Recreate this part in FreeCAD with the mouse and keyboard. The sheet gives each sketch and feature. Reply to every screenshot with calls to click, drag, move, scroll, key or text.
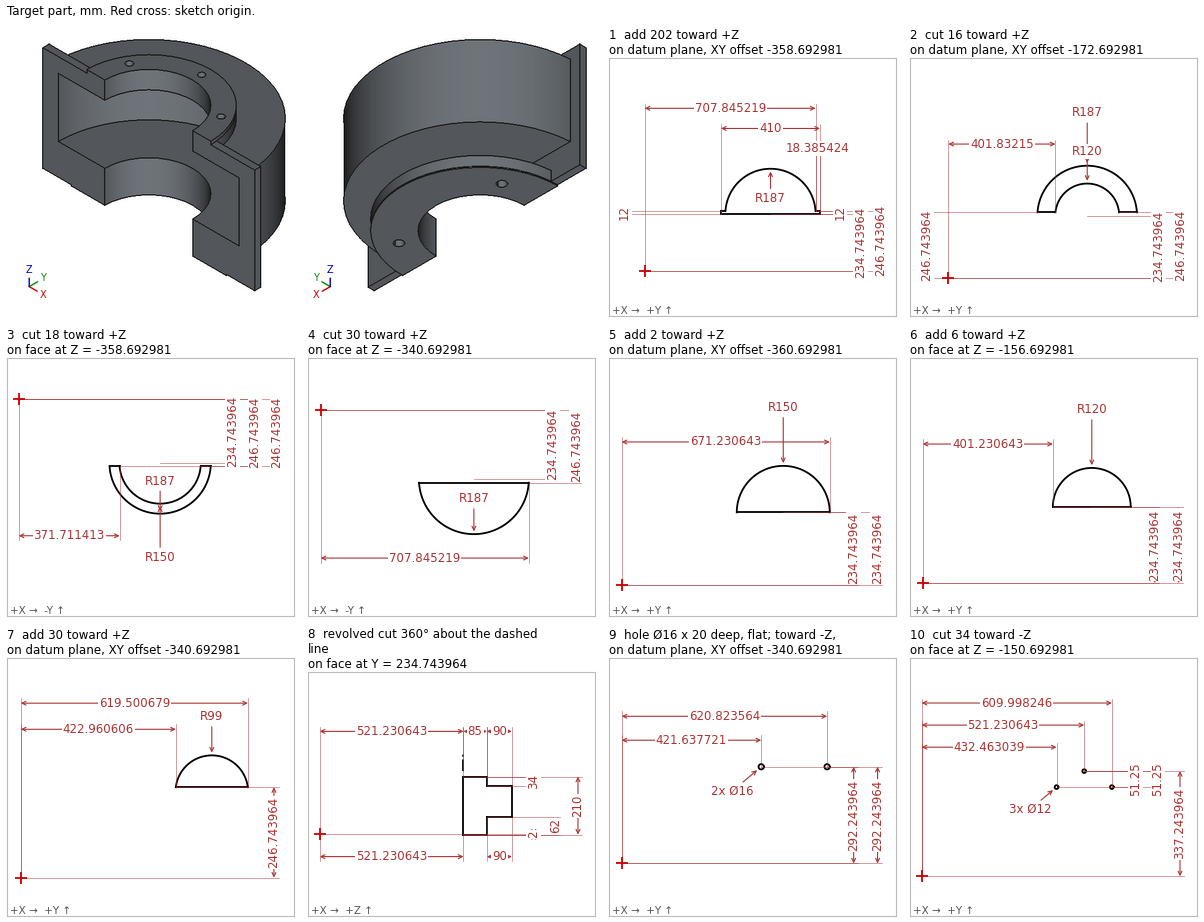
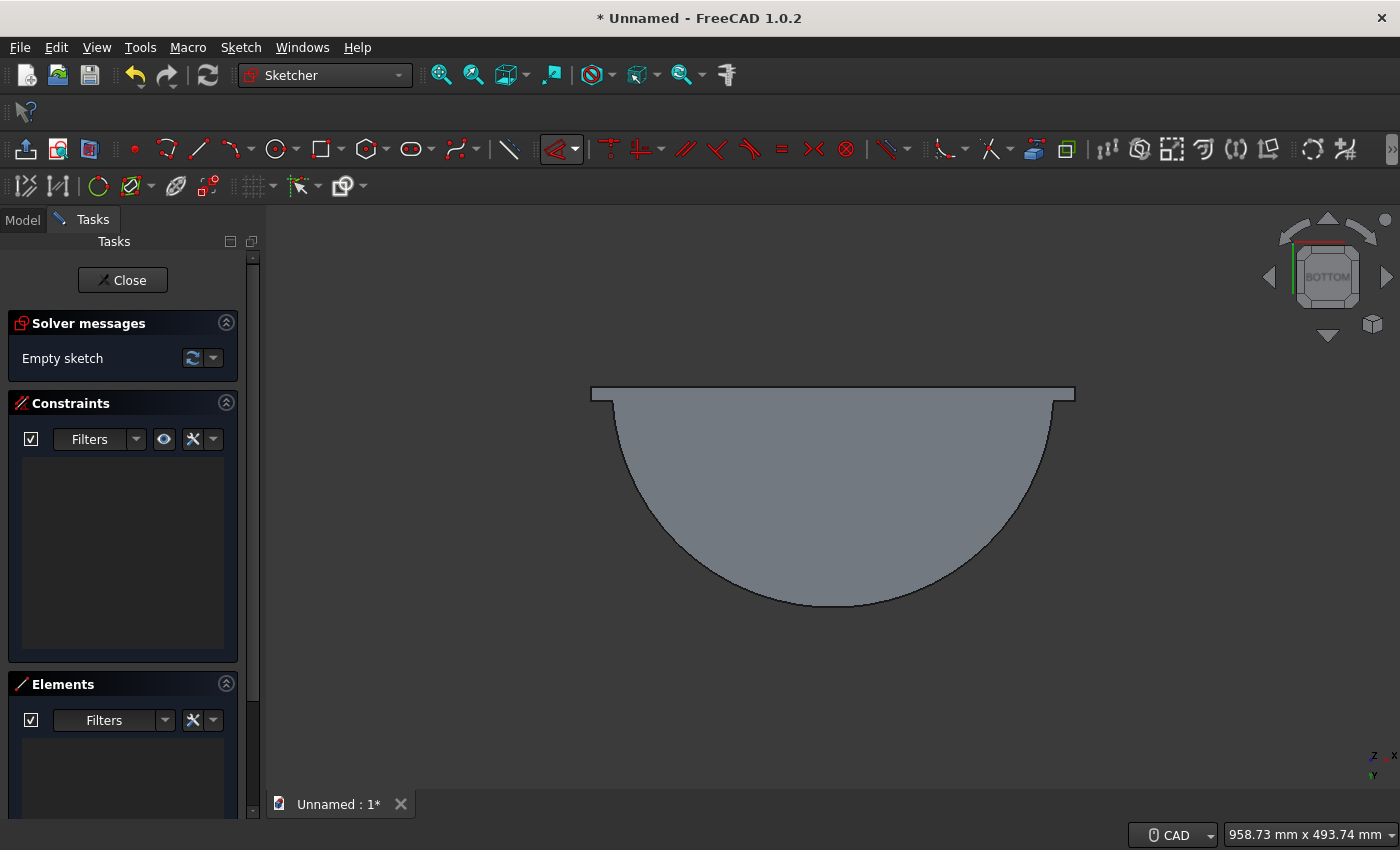
scroll(1028, 761, down, 2)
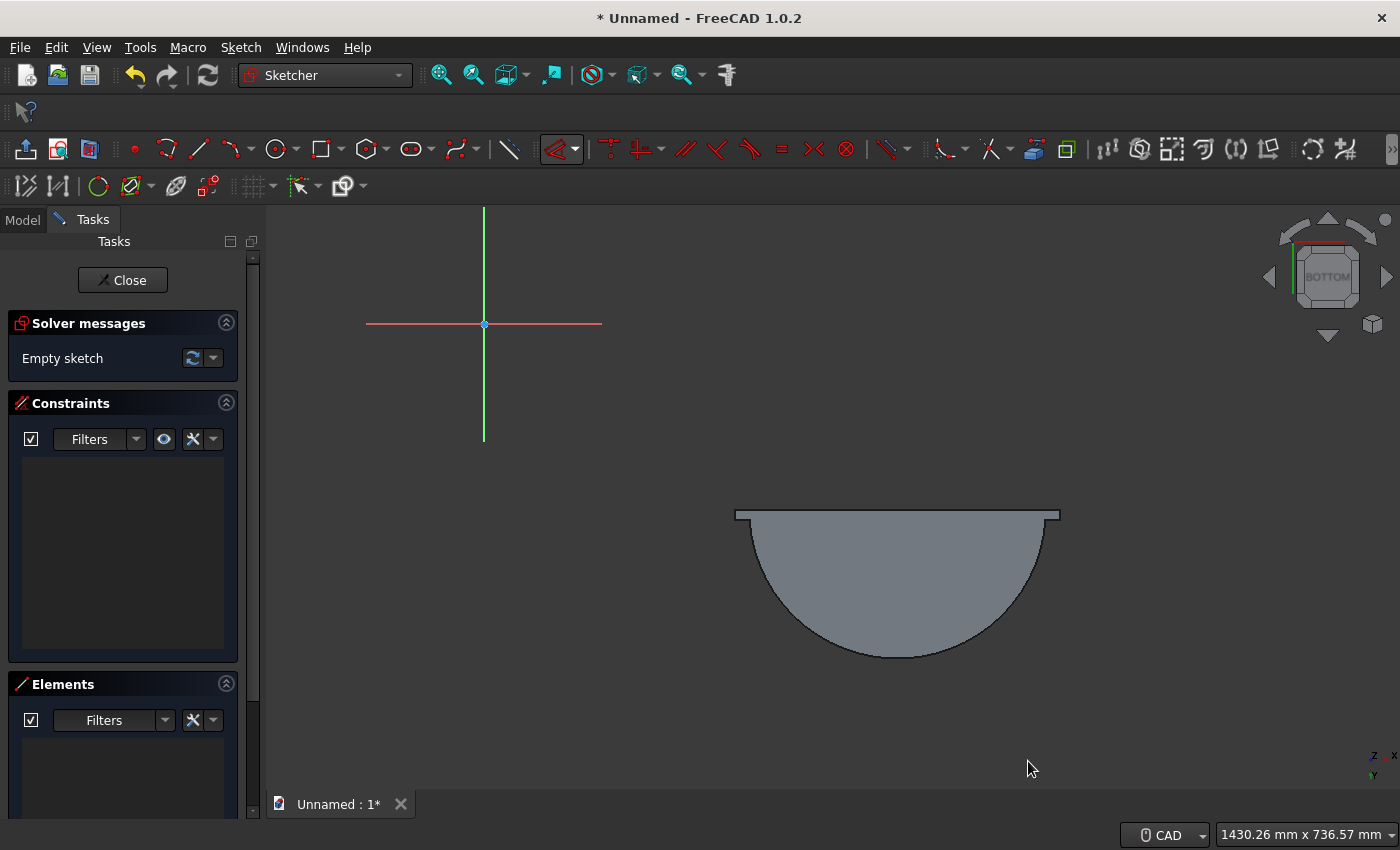
key(g)
key(l)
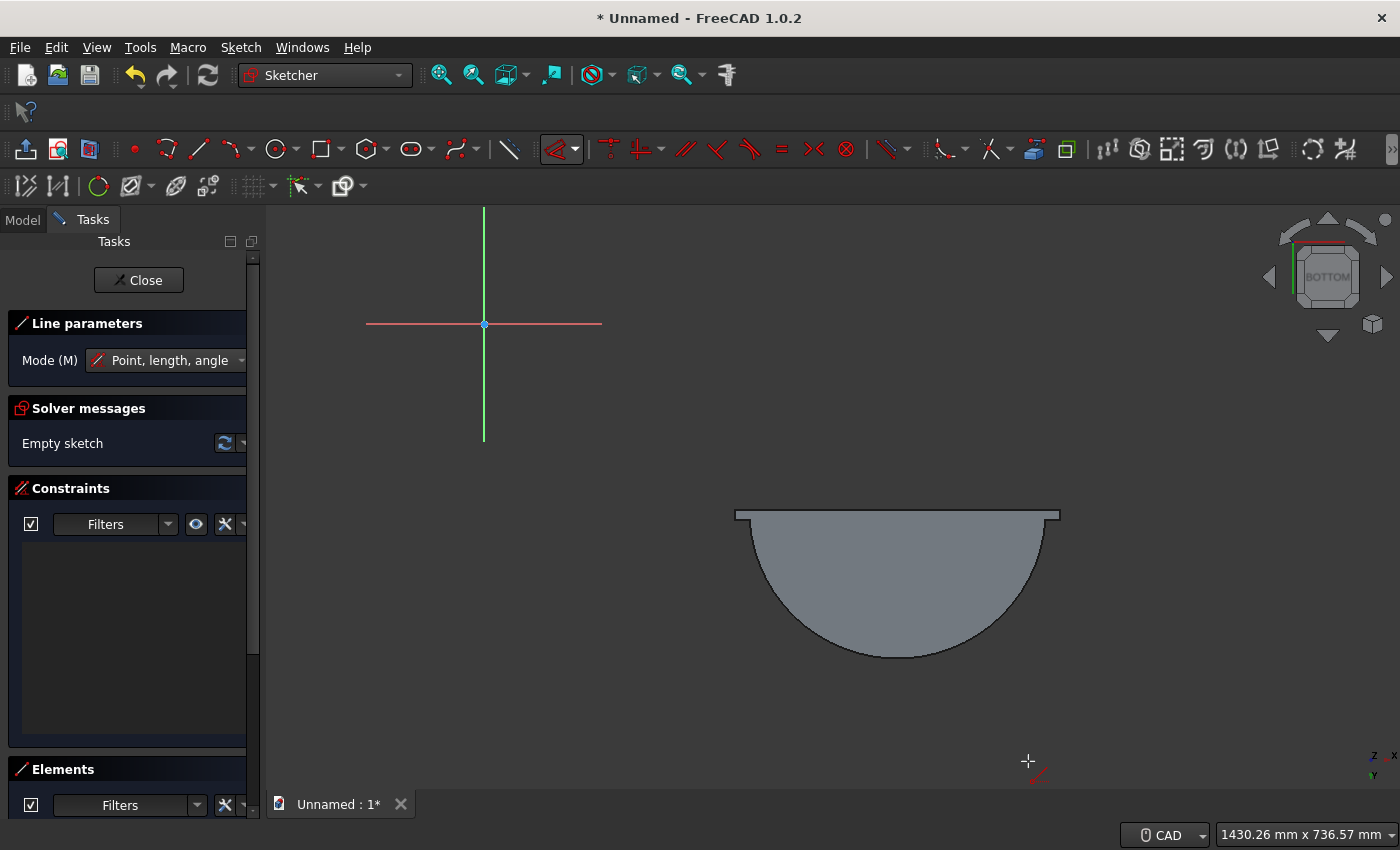
click(779, 520)
click(750, 520)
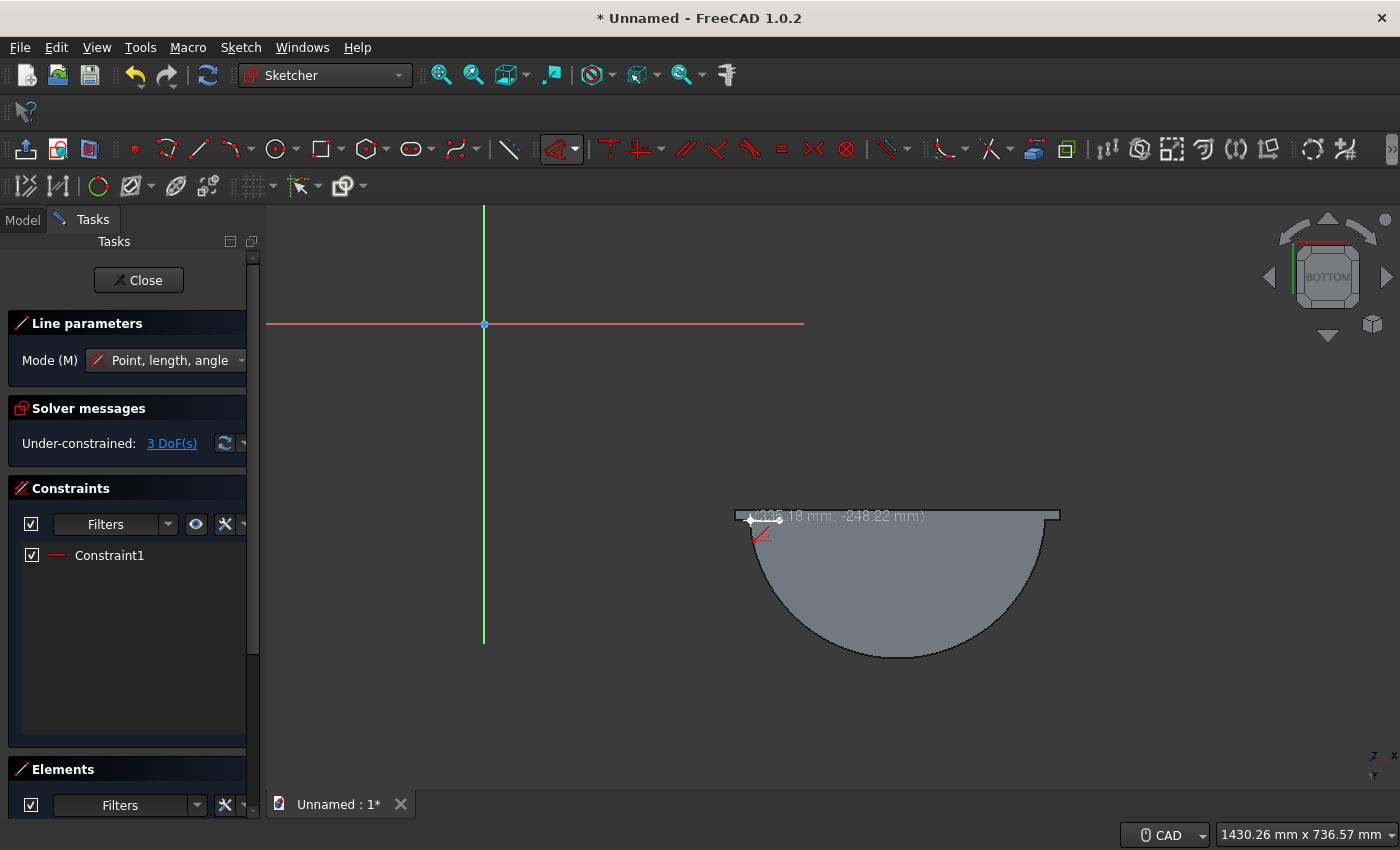
click(1045, 520)
click(1016, 520)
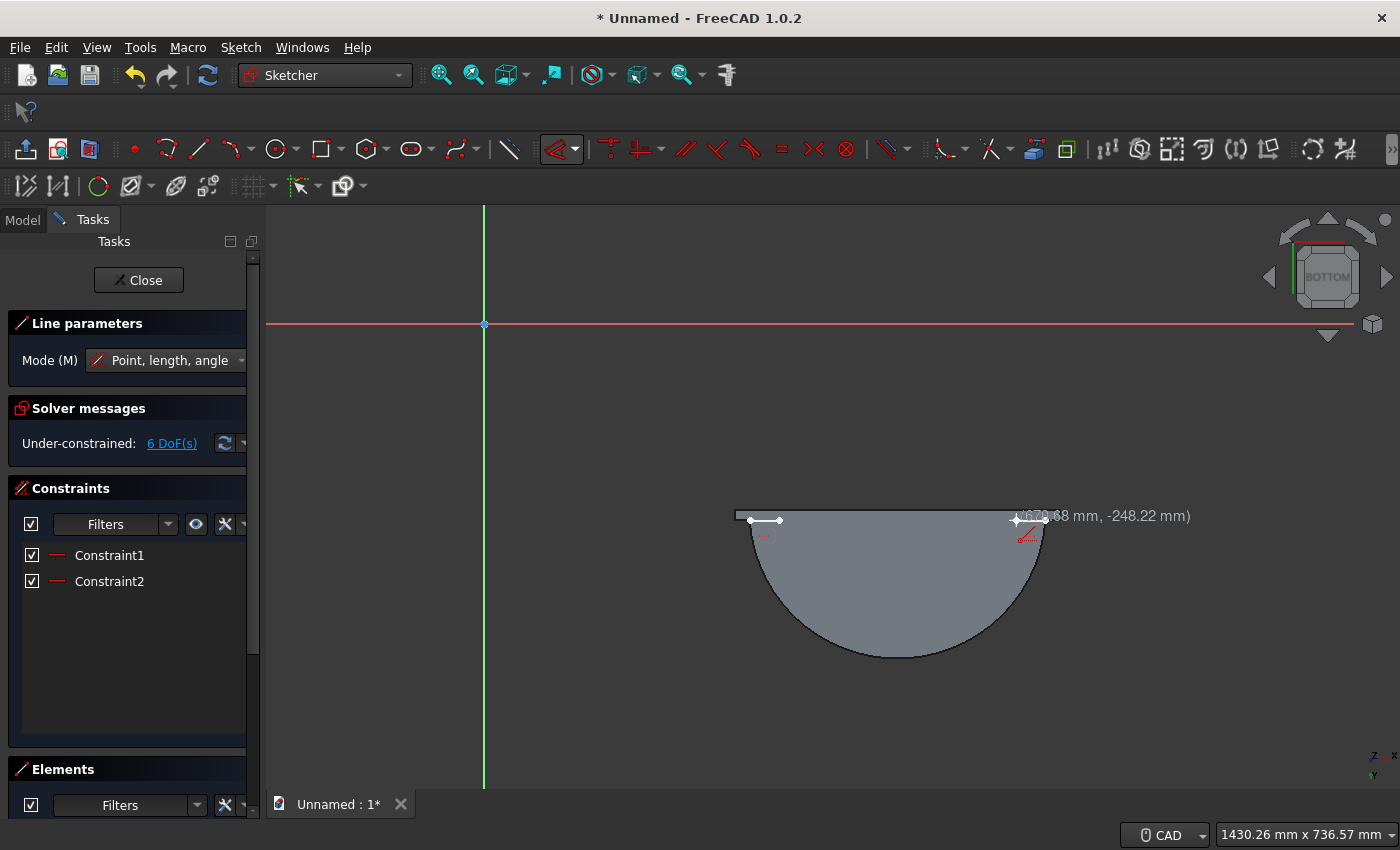
click(232, 150)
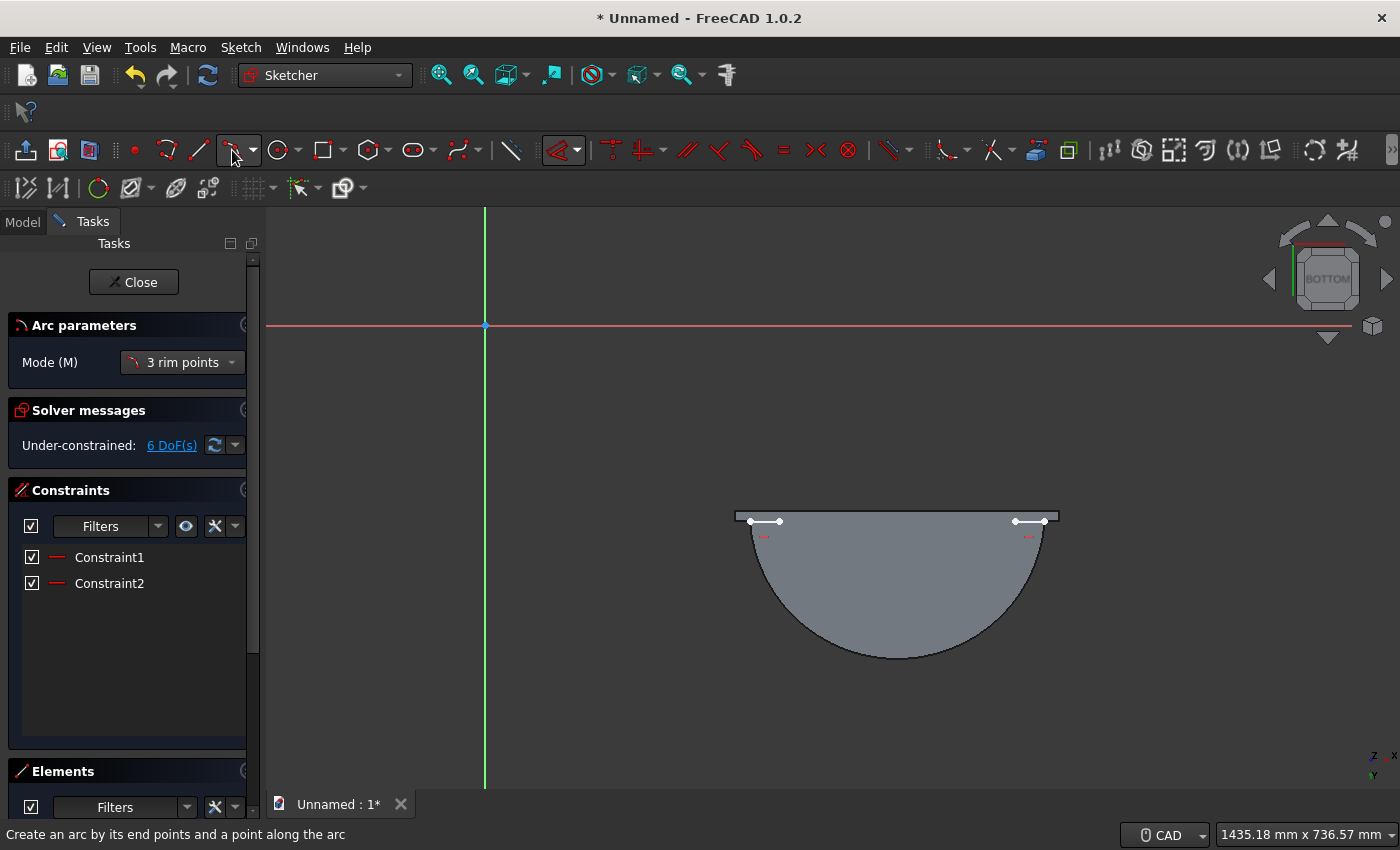
click(750, 522)
click(1044, 522)
click(897, 659)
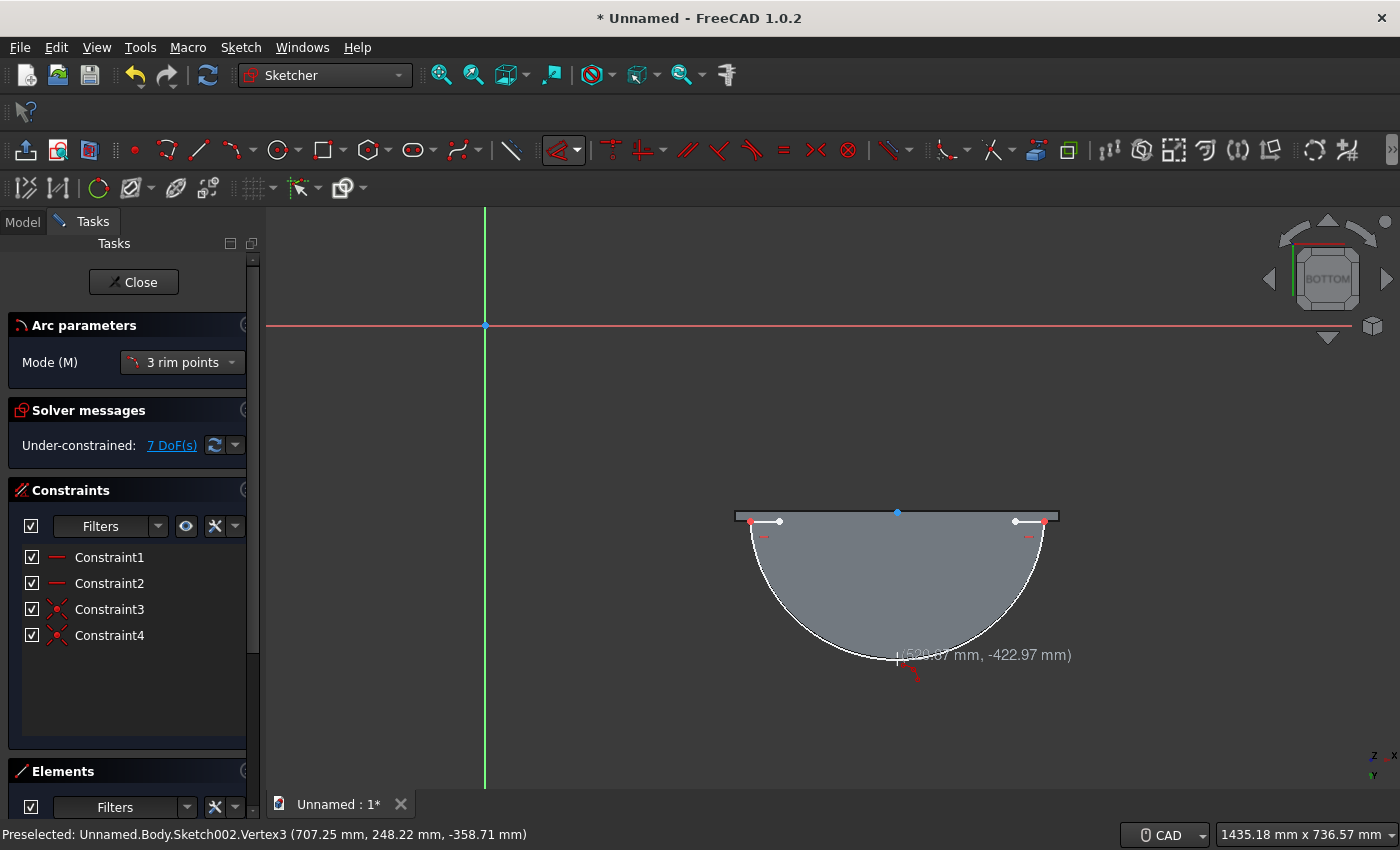
click(1015, 522)
click(779, 522)
click(897, 630)
key(Escape)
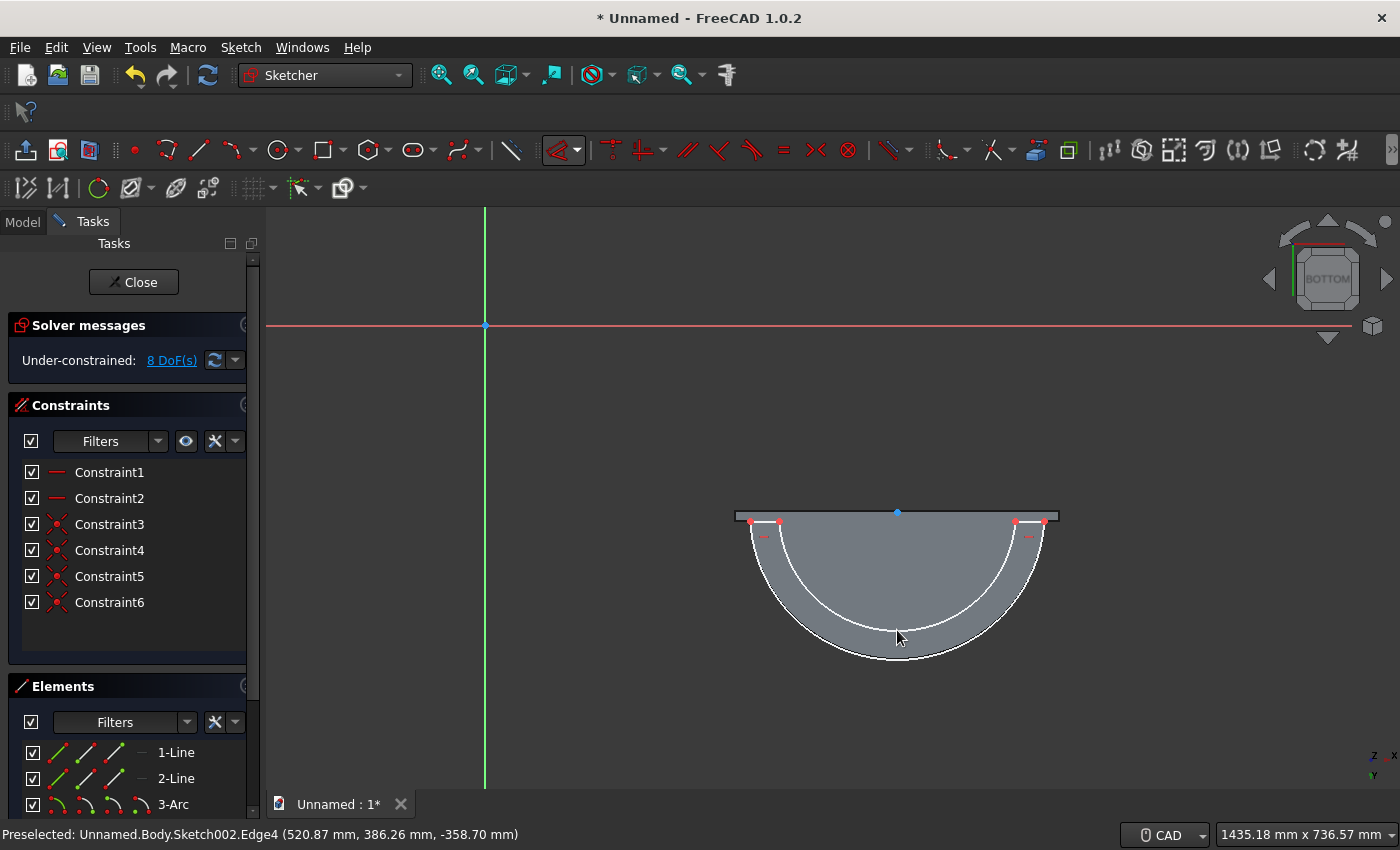
click(814, 634)